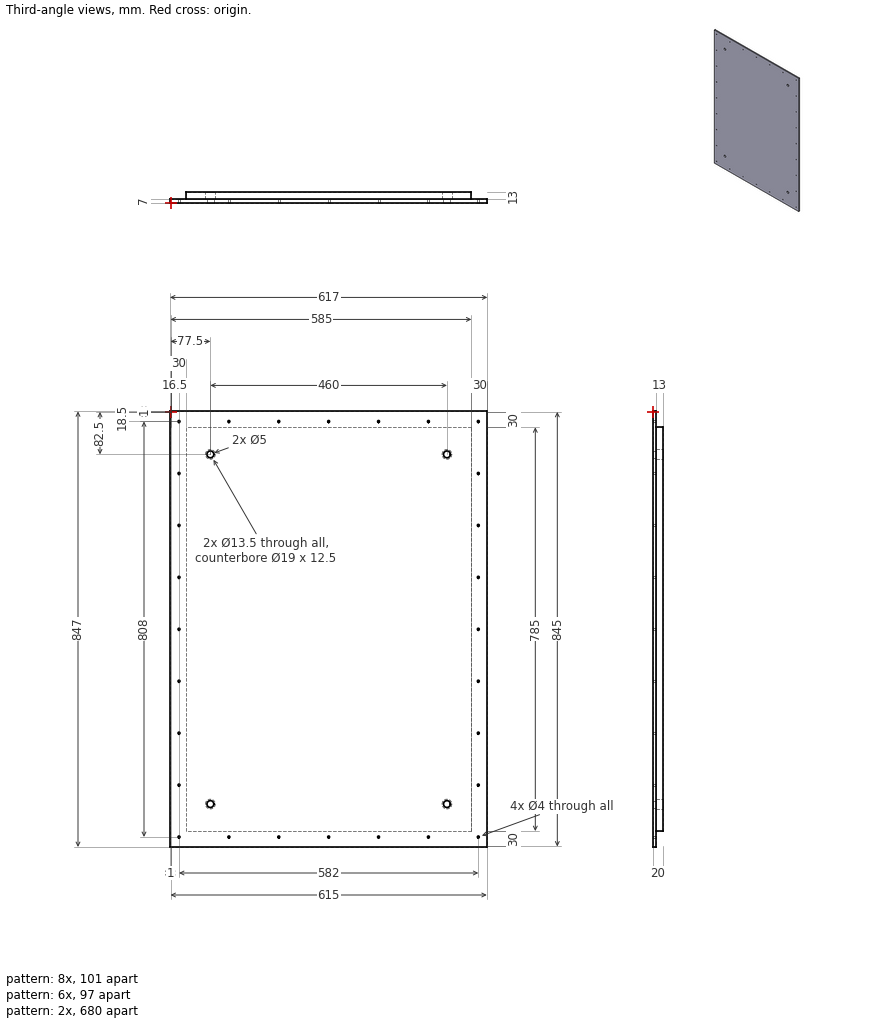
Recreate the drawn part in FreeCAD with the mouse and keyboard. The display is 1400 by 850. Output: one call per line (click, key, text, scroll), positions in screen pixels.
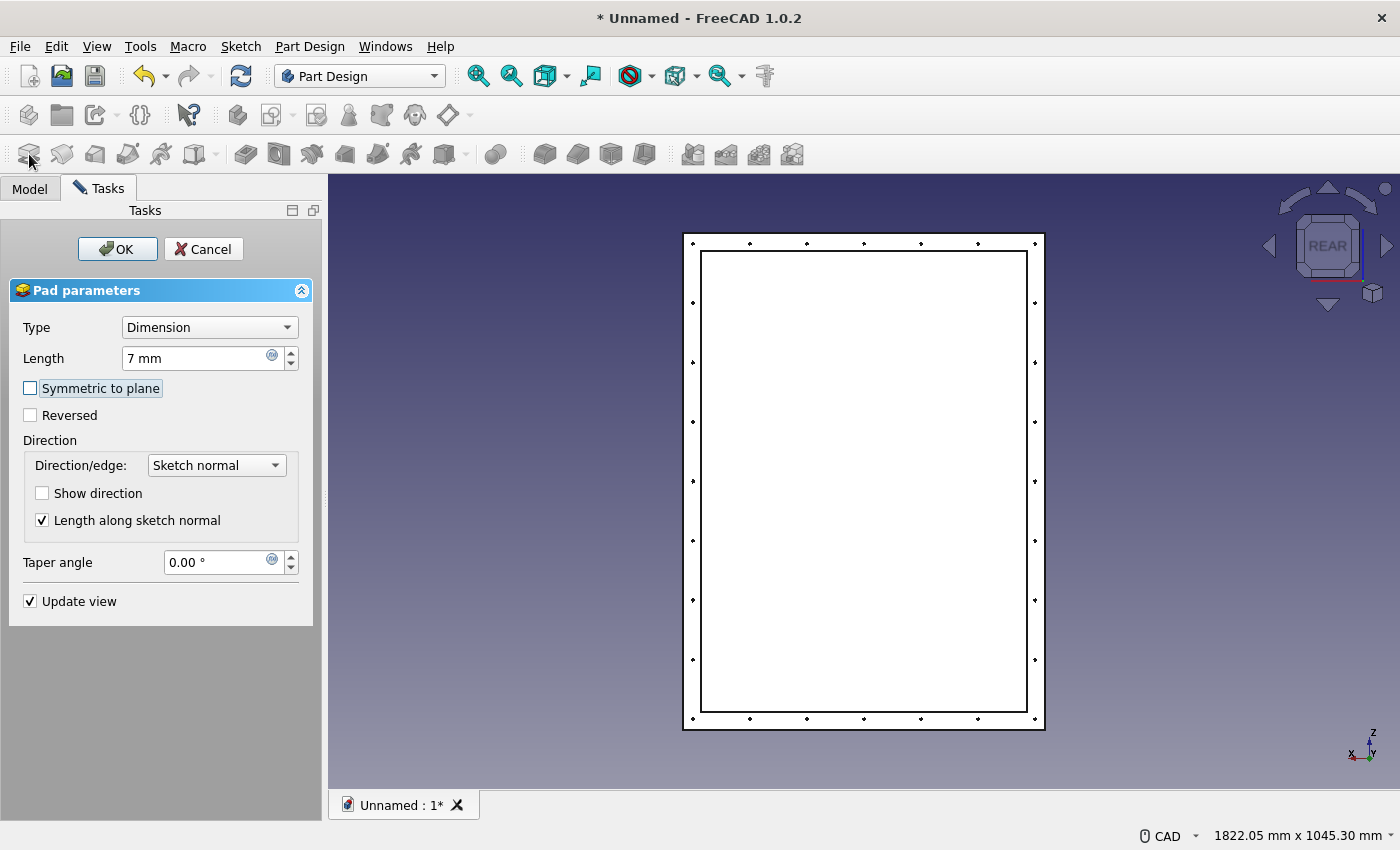
click(31, 415)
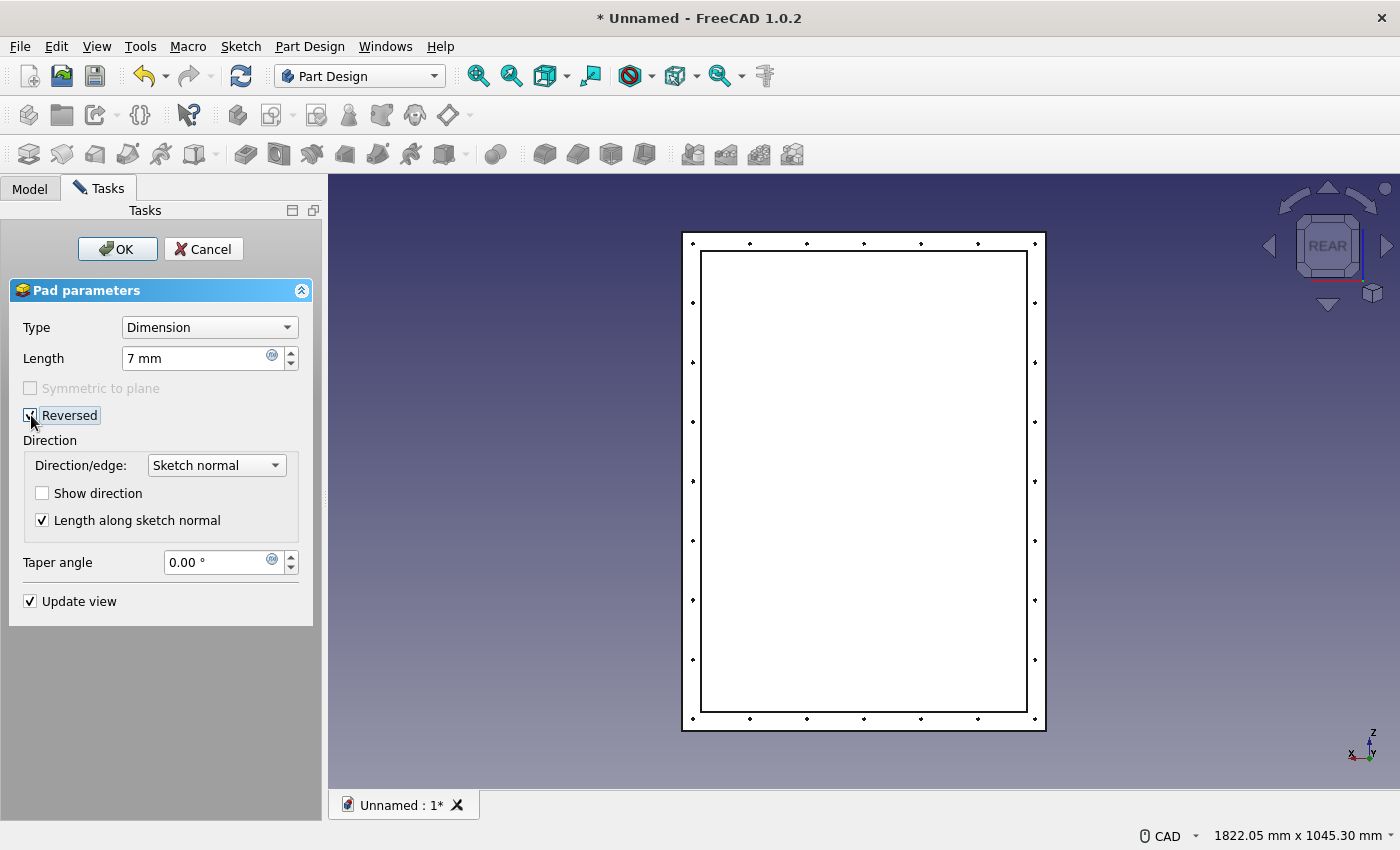
click(118, 249)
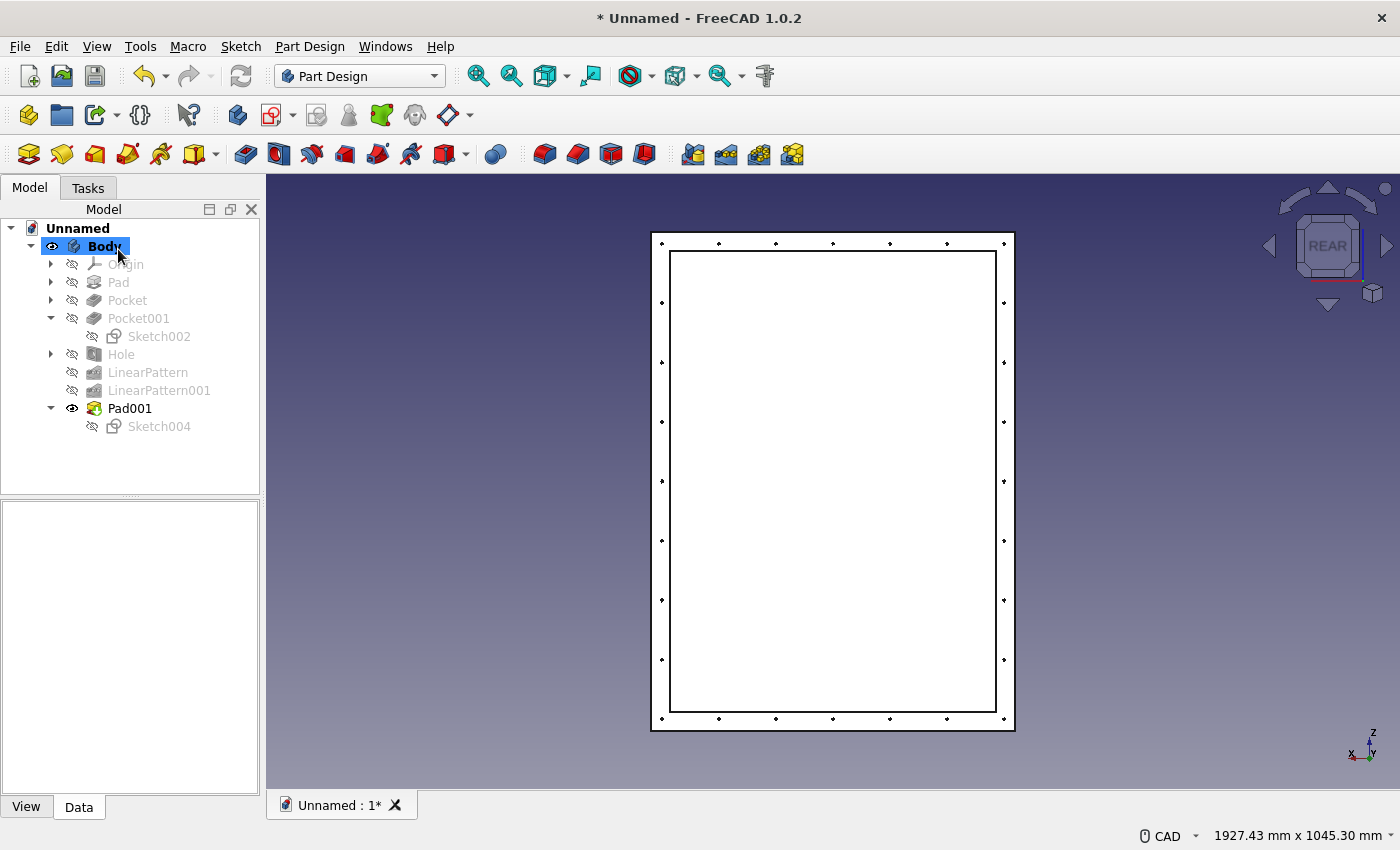
click(833, 415)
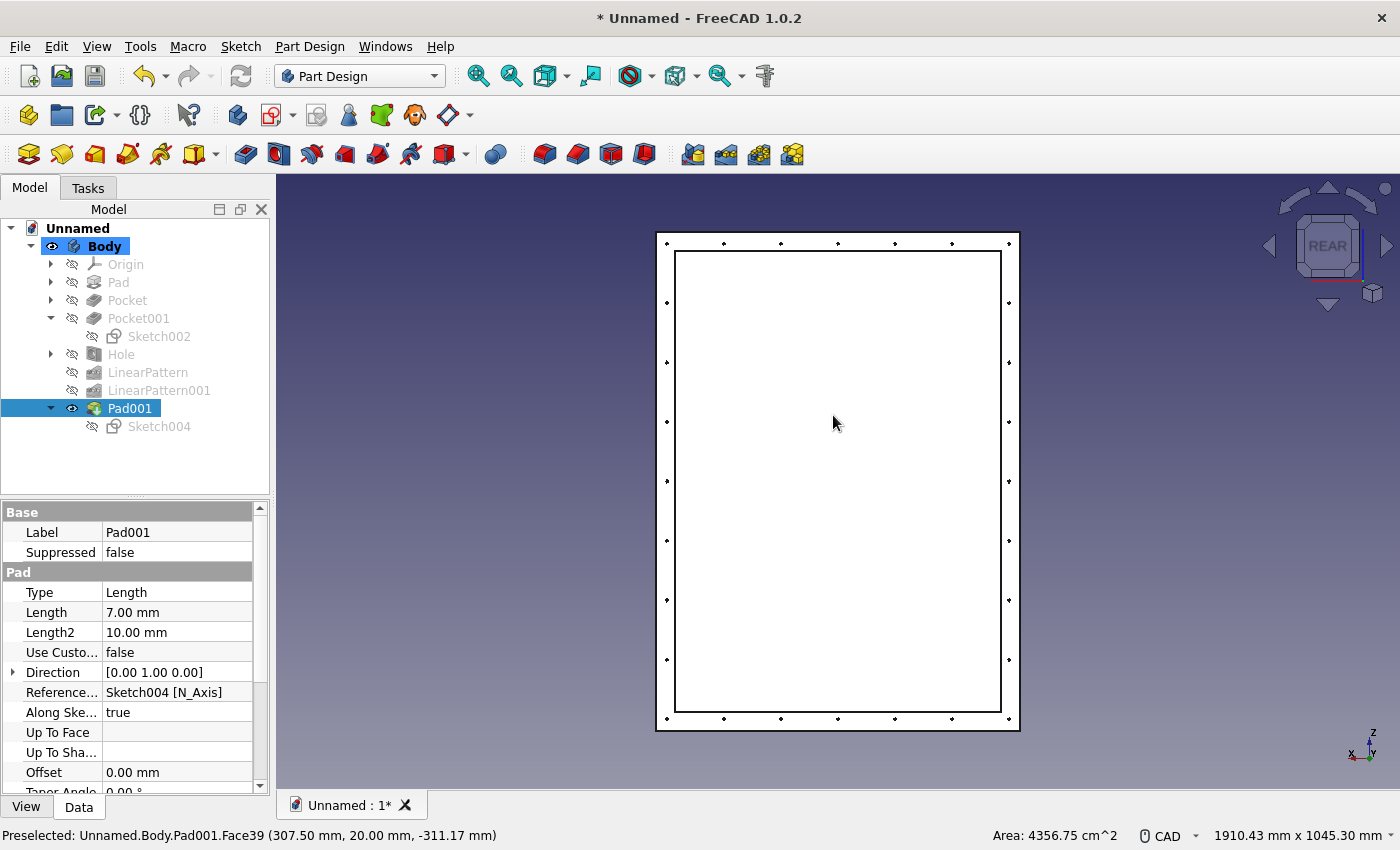
click(270, 116)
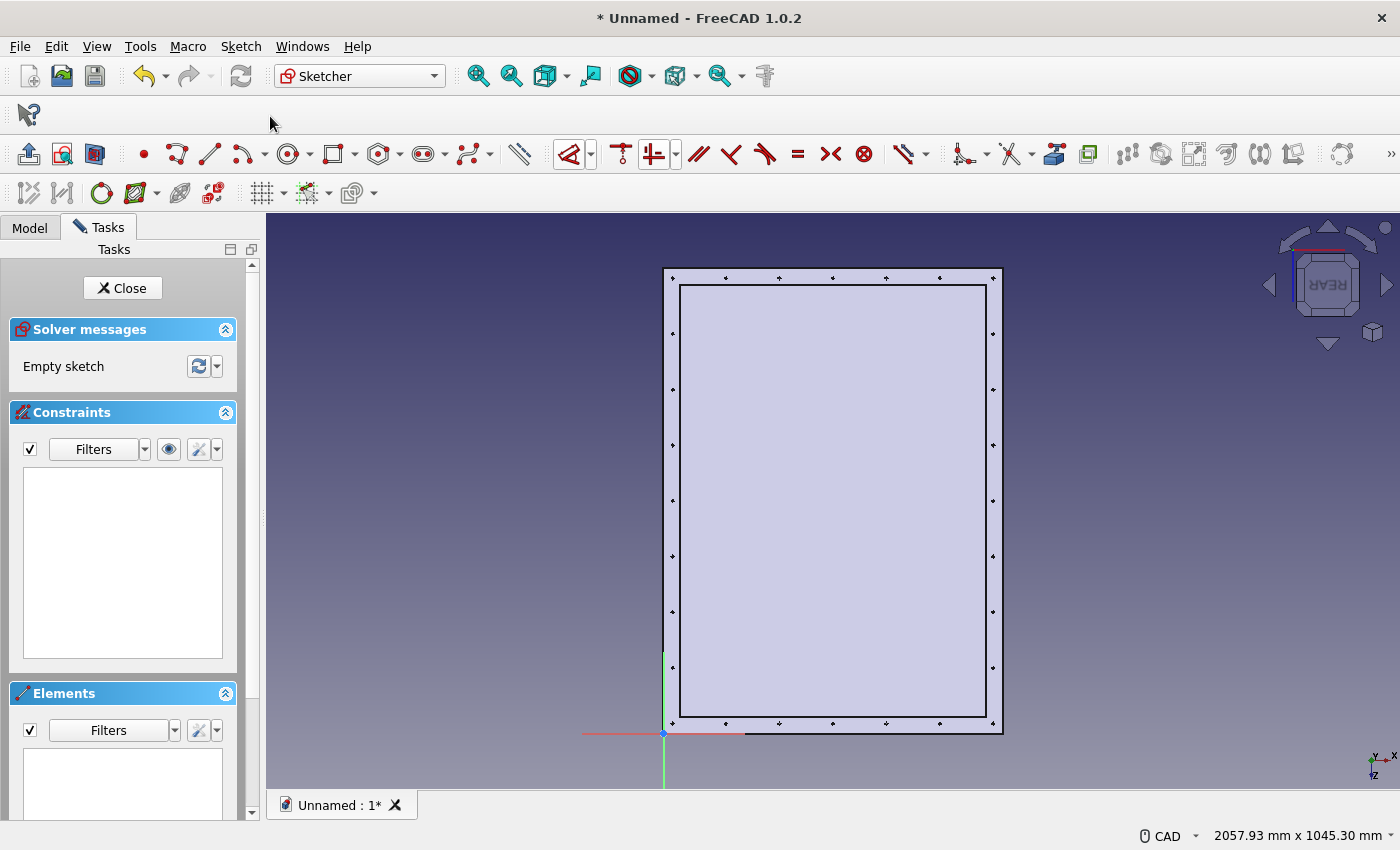
scroll(851, 761, up, 4)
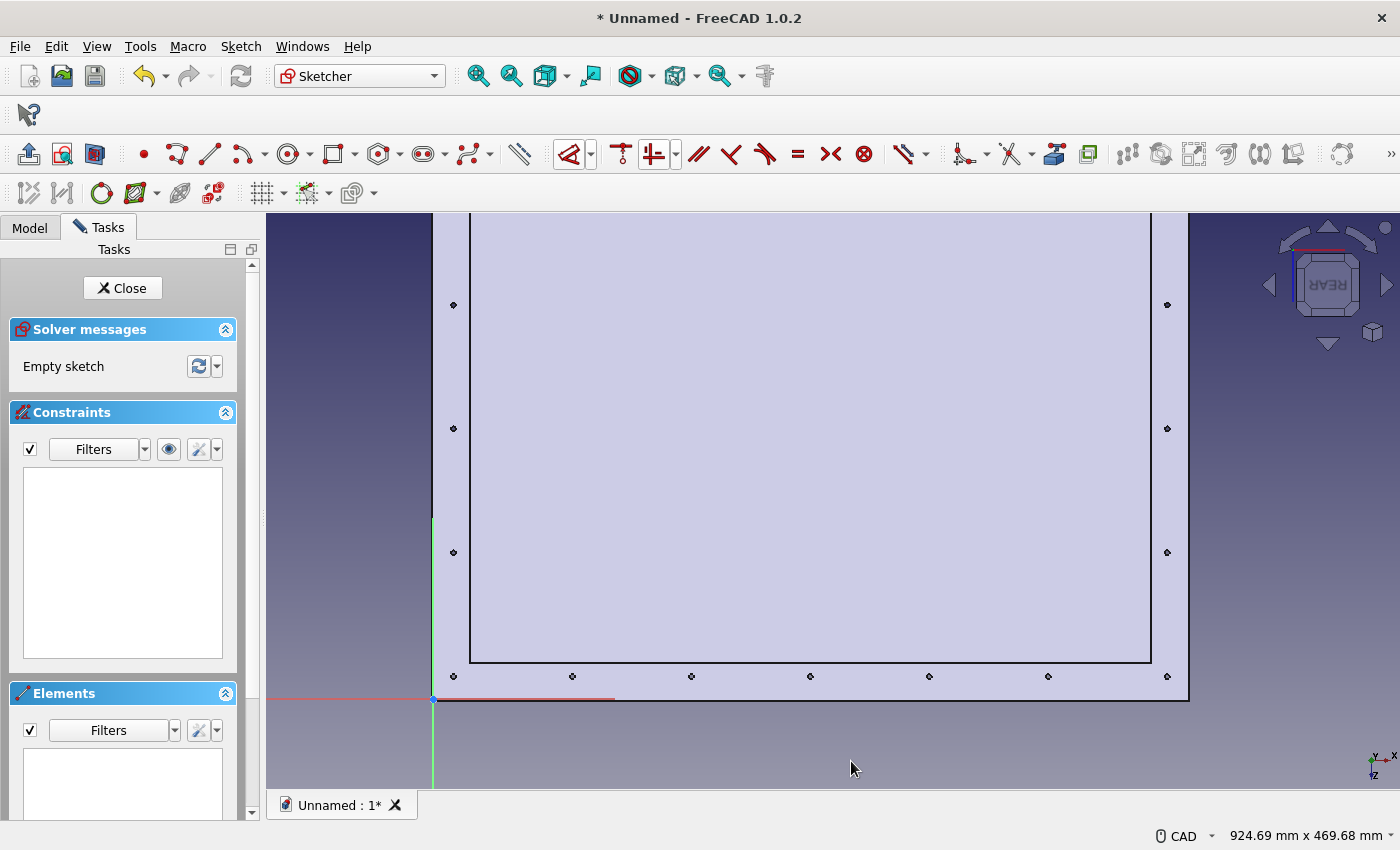
click(288, 154)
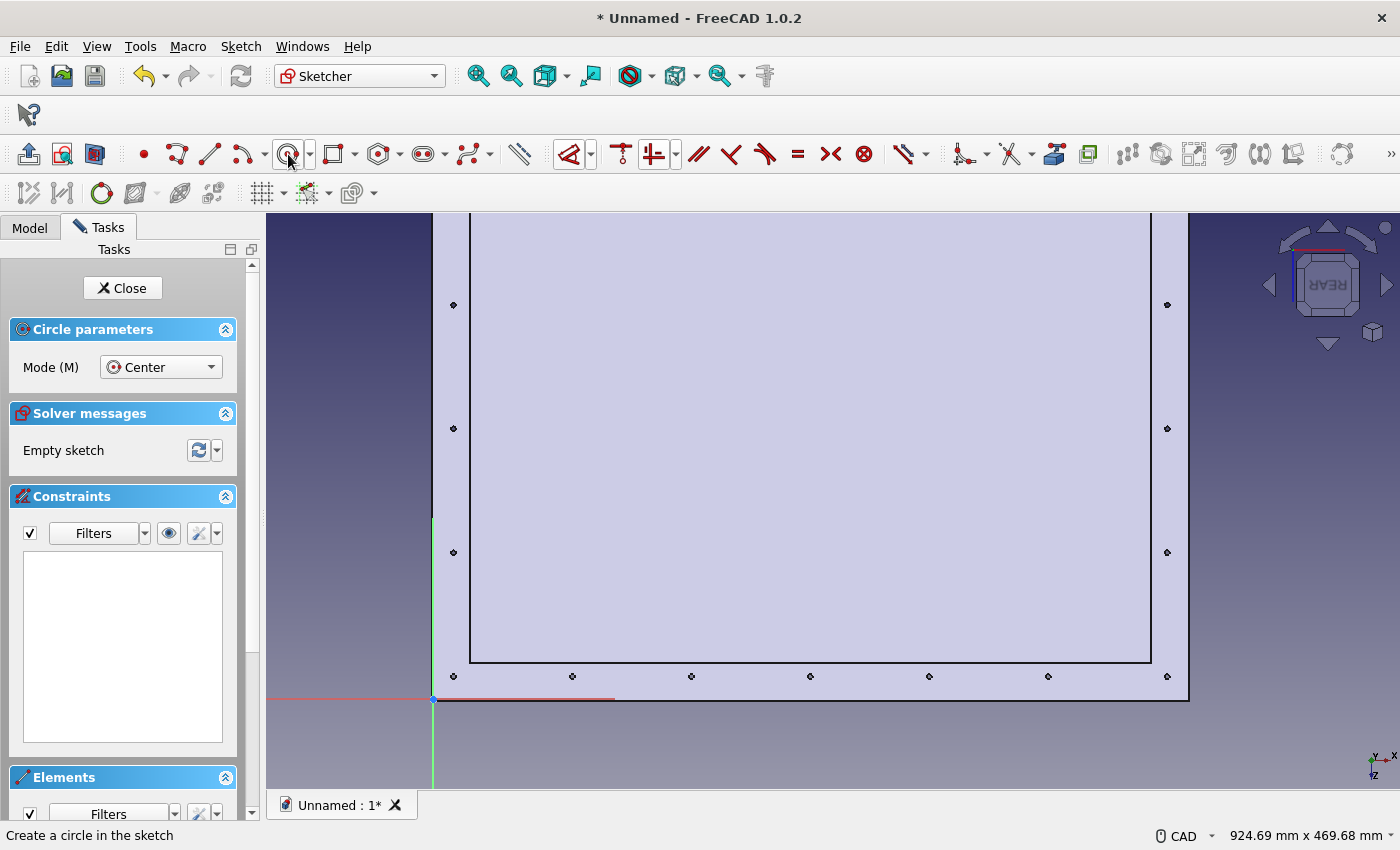
scroll(528, 598, up, 11)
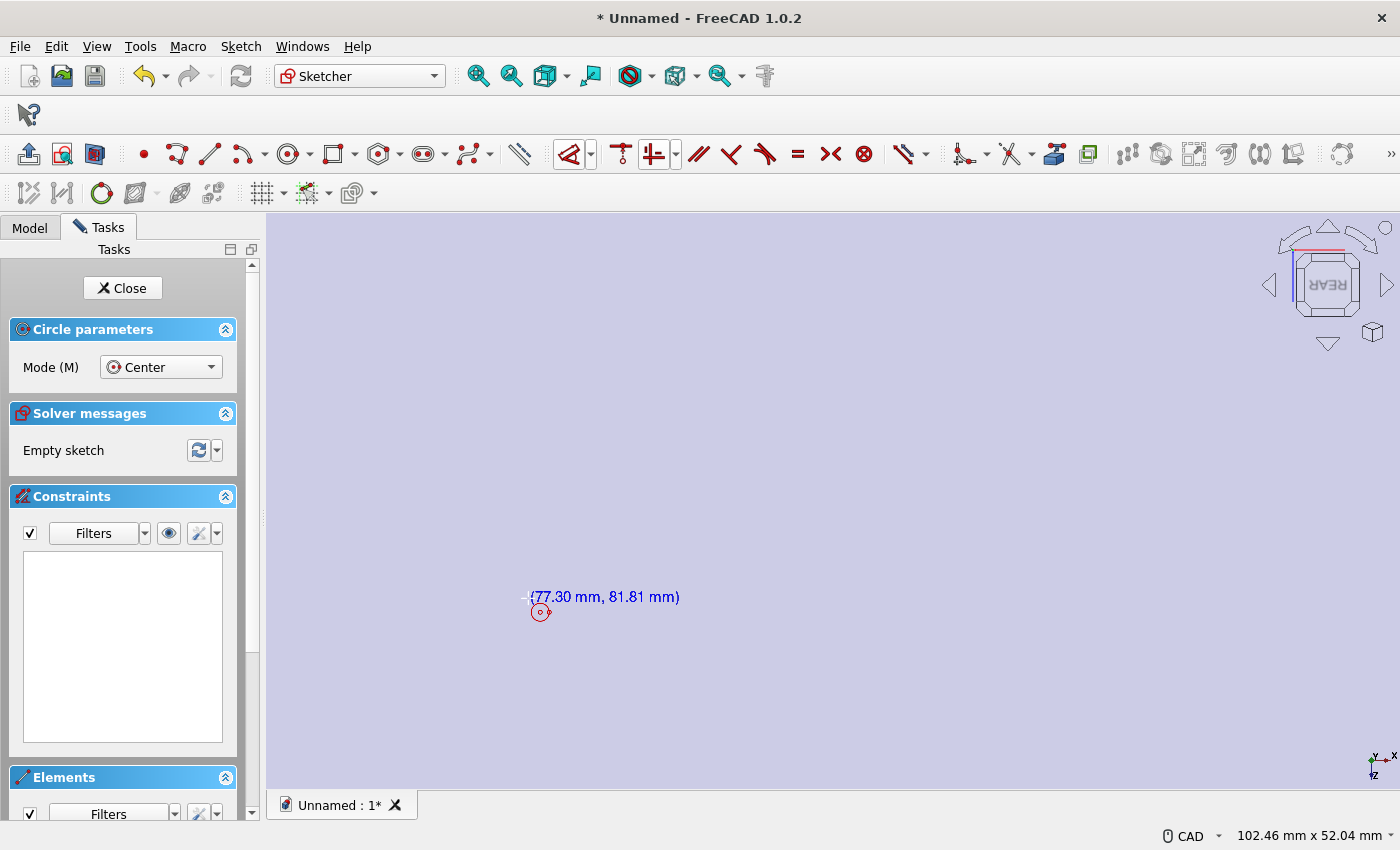
scroll(528, 434, down, 11)